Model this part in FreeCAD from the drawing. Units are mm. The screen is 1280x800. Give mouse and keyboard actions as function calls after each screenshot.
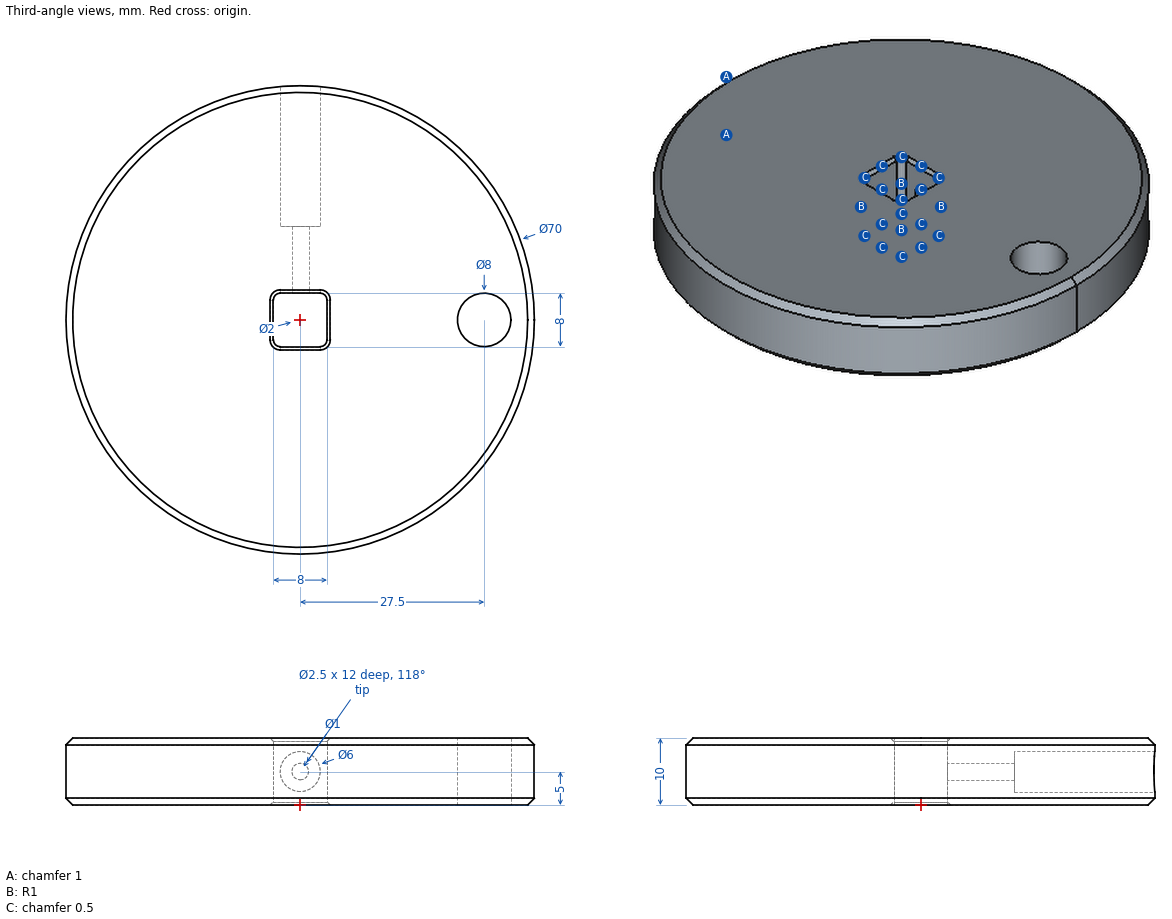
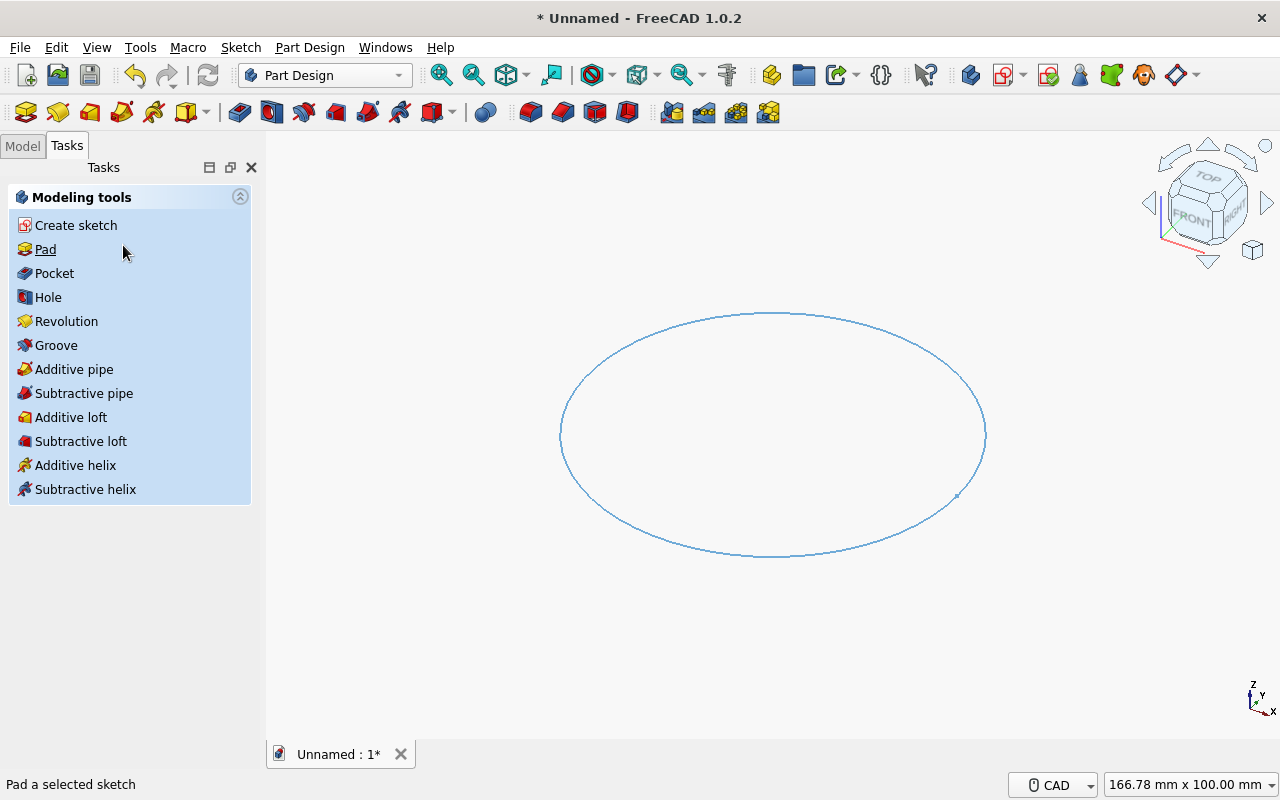
click(26, 112)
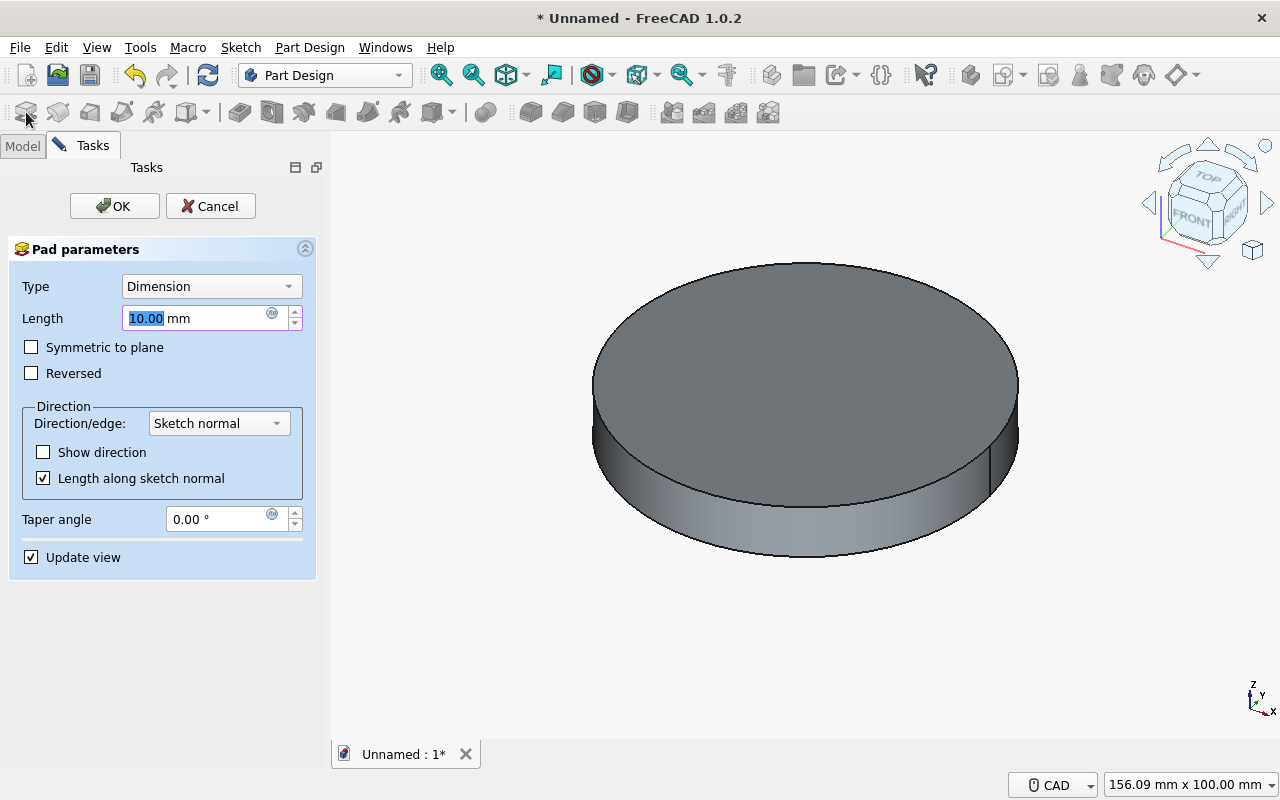
text(10)
key(Tab)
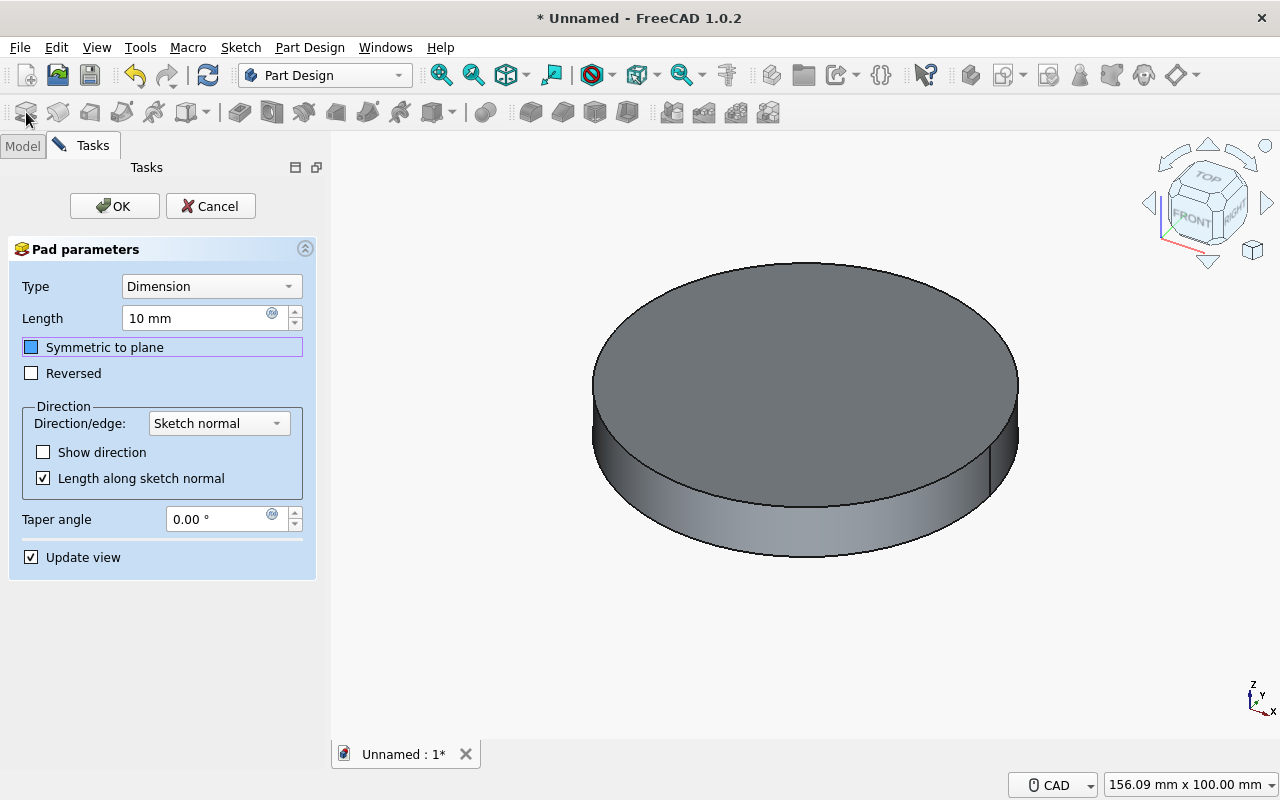
click(115, 206)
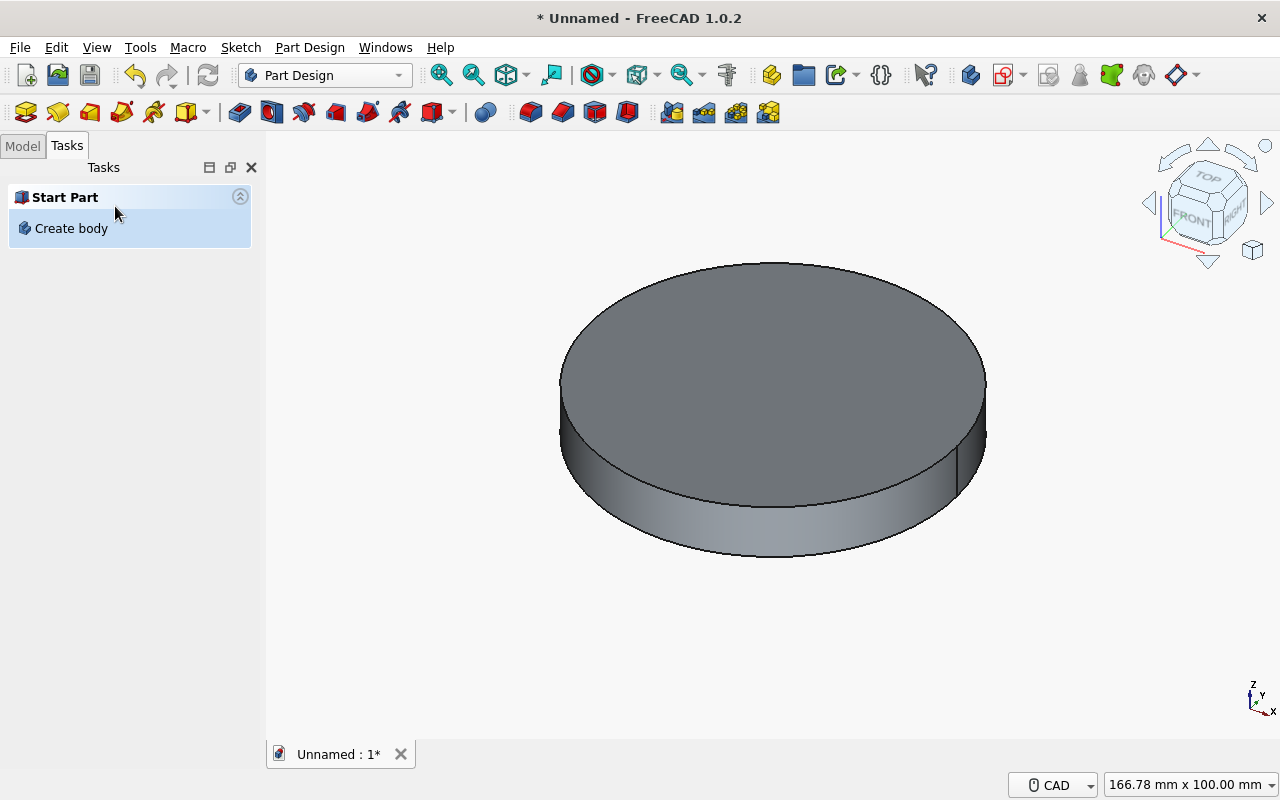
click(561, 397)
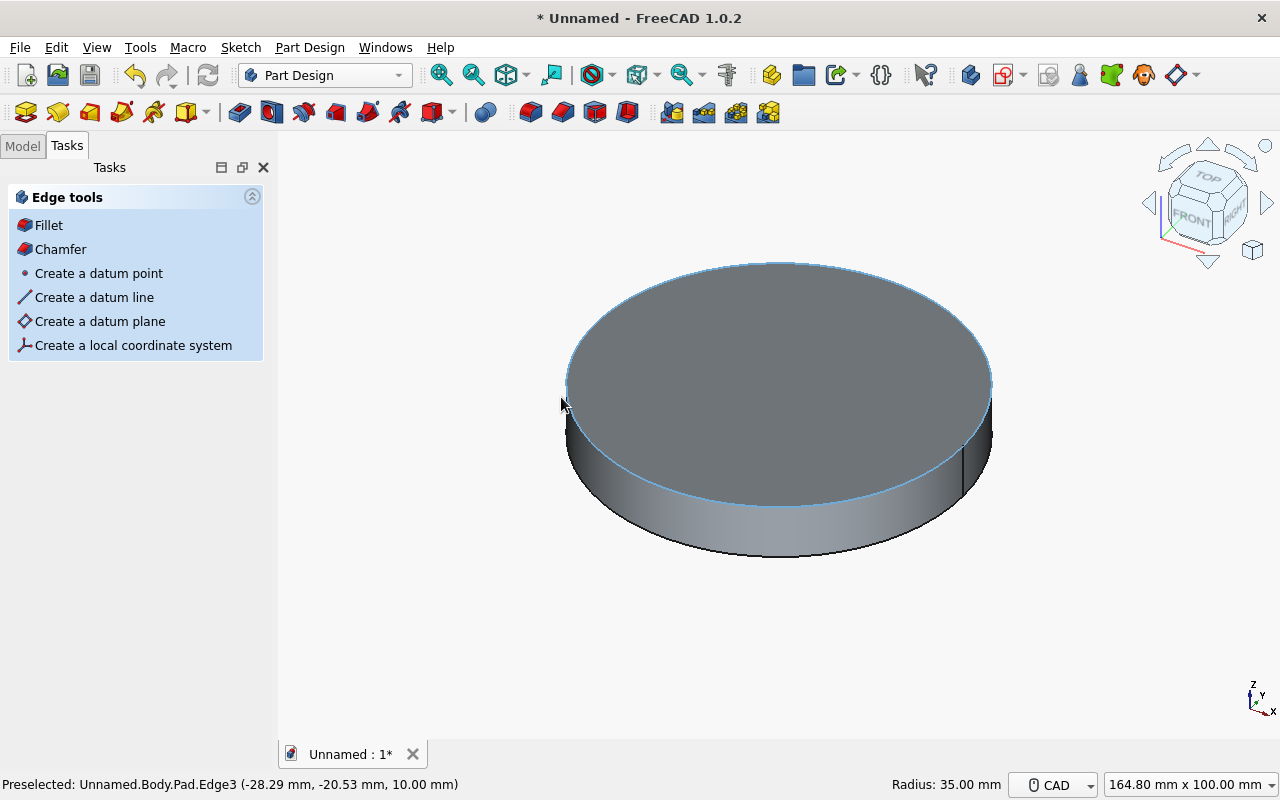
key(0)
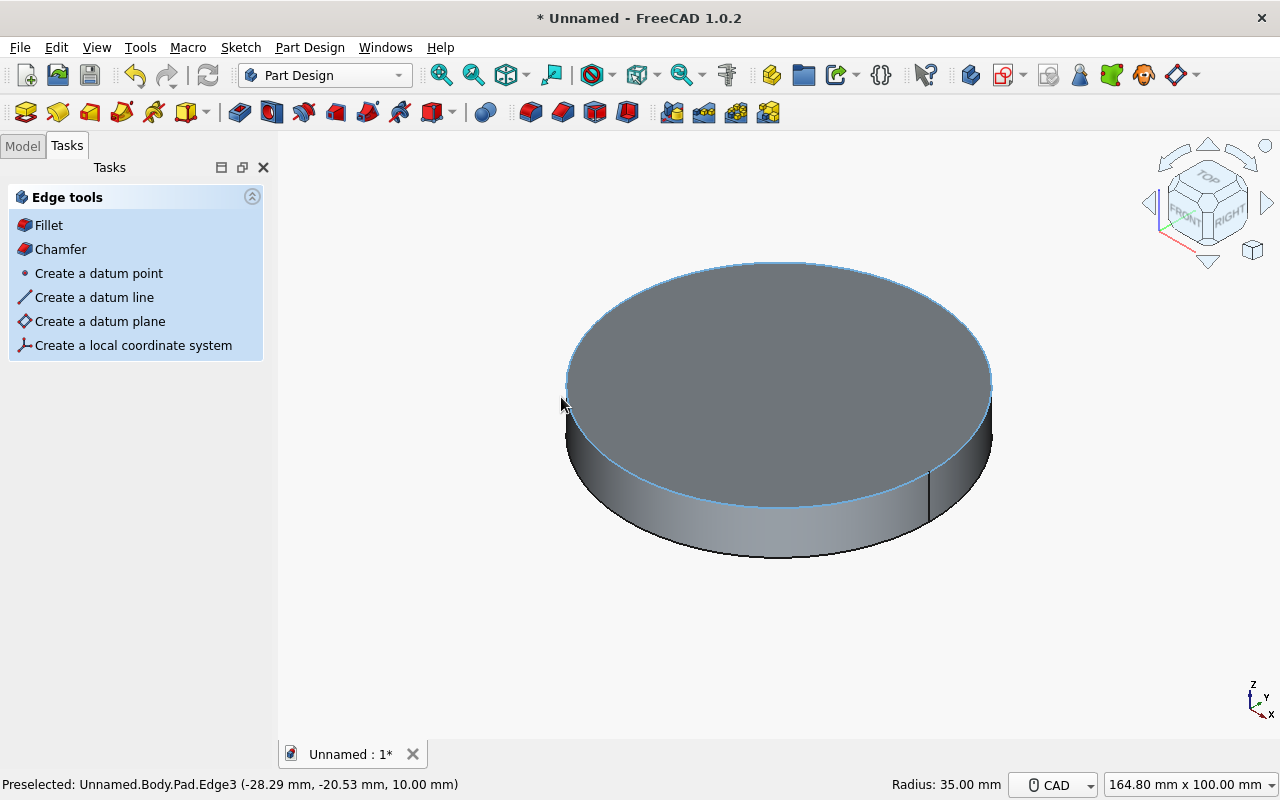
key(2)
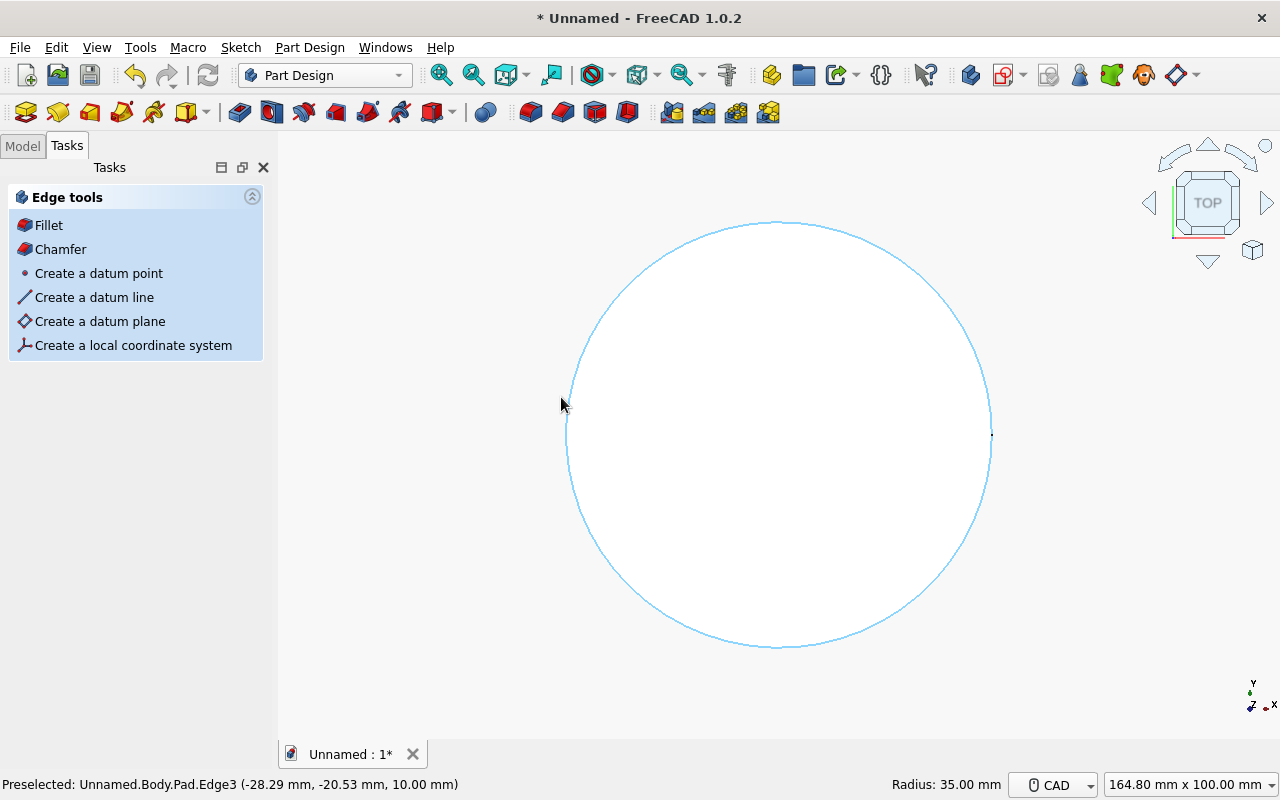
key(1)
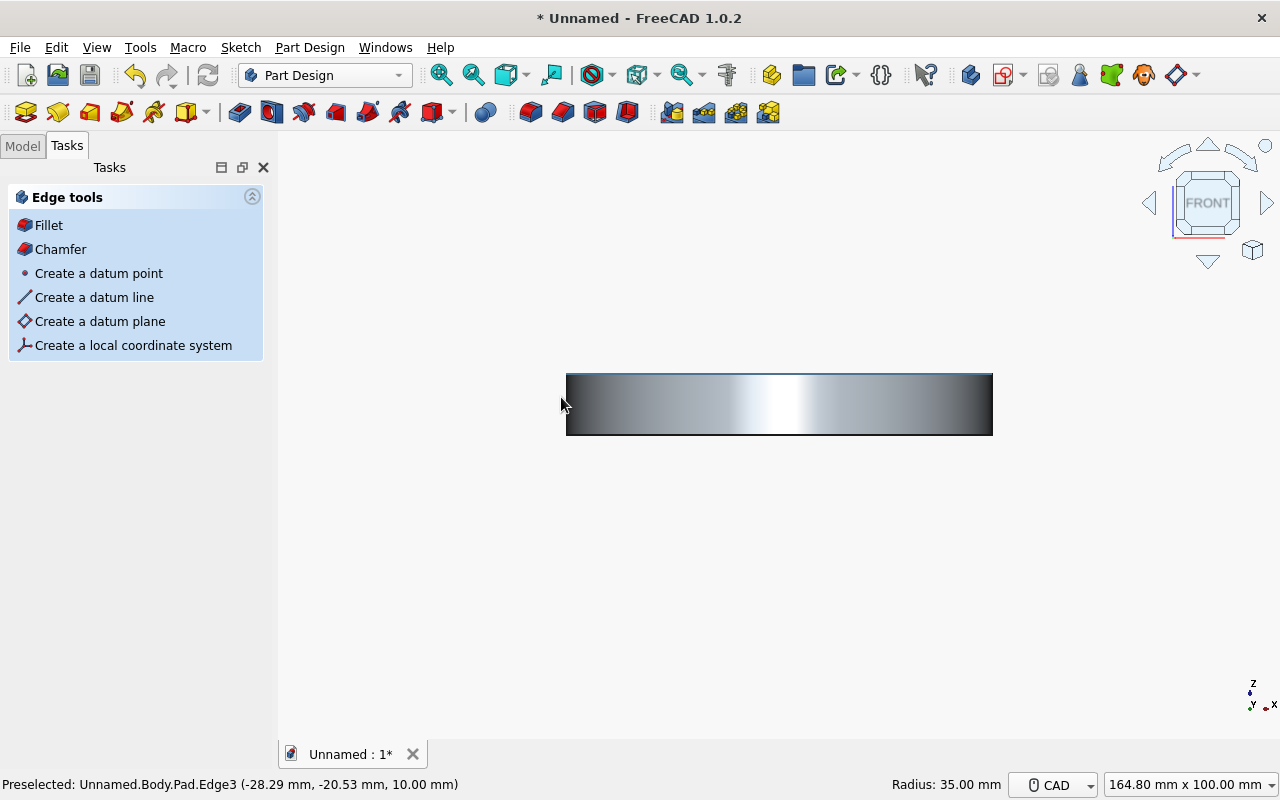
click(442, 76)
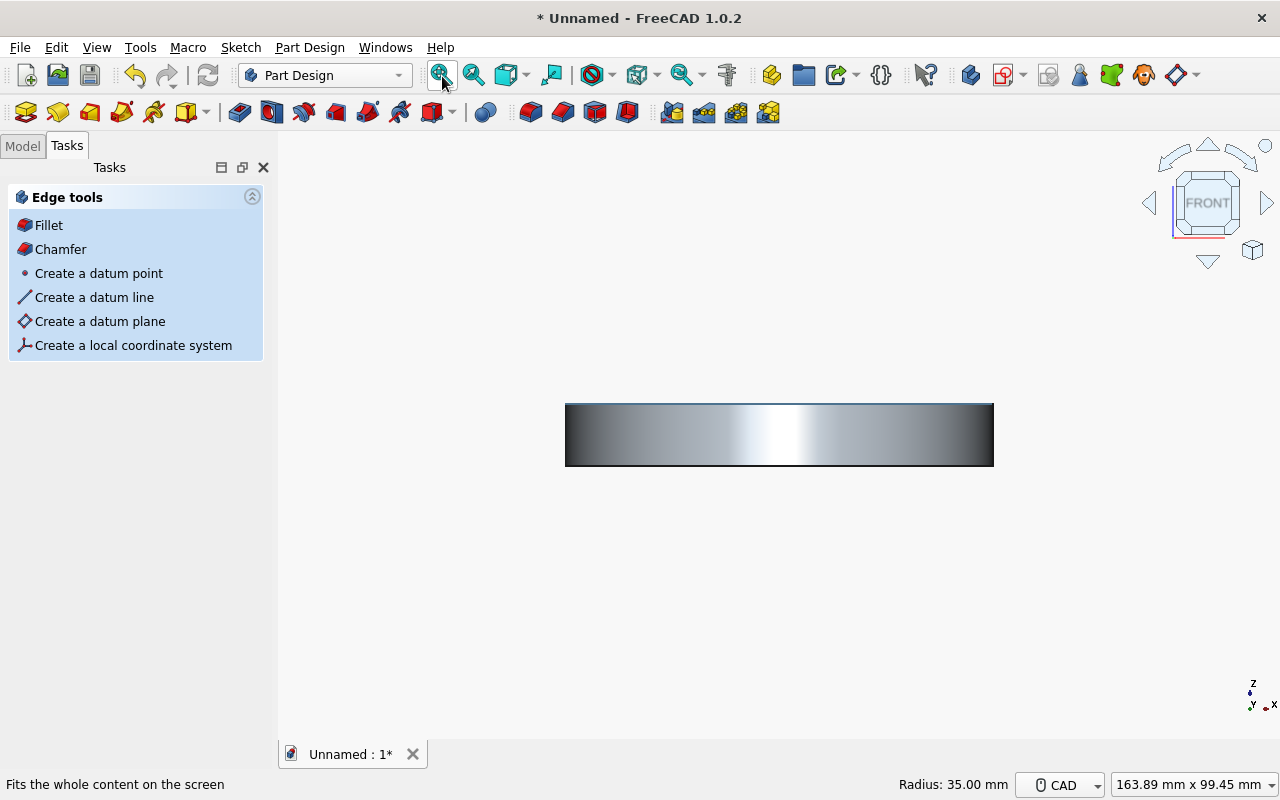
click(606, 465, ctrl)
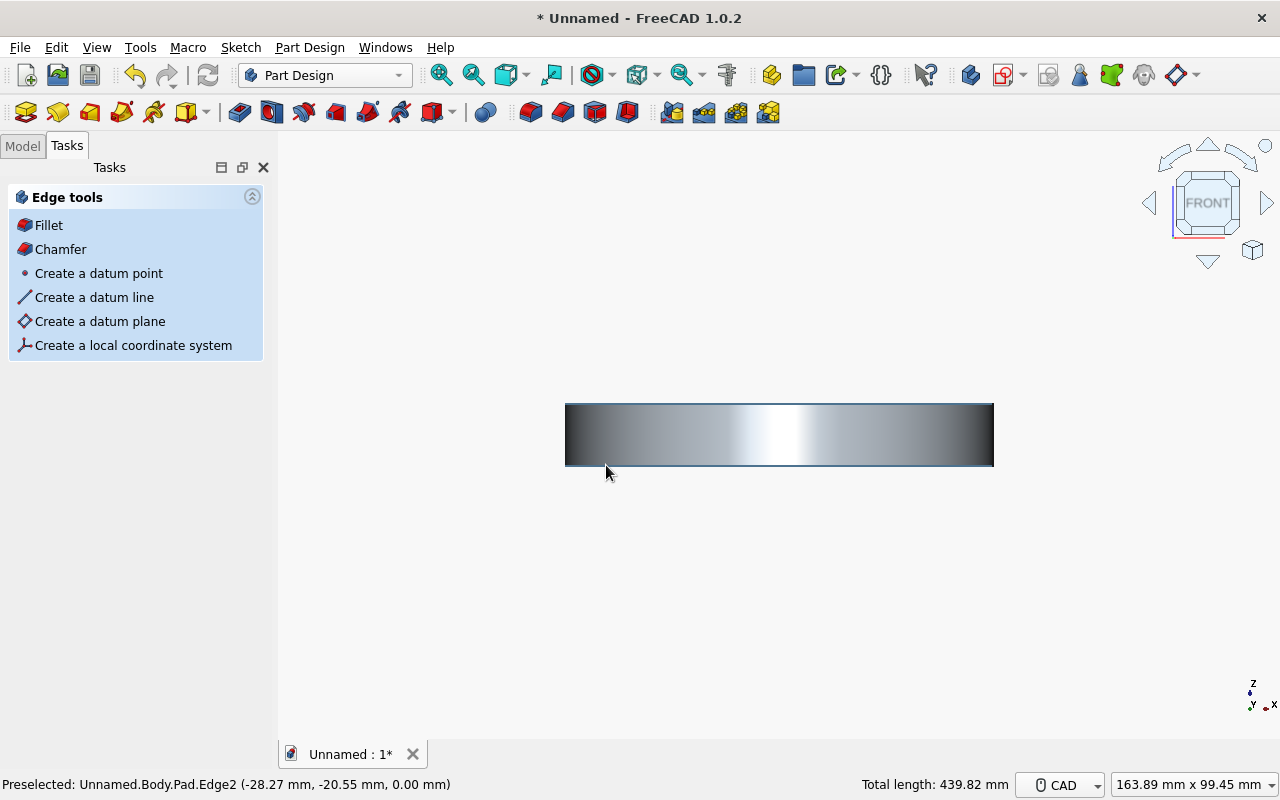
click(564, 112)